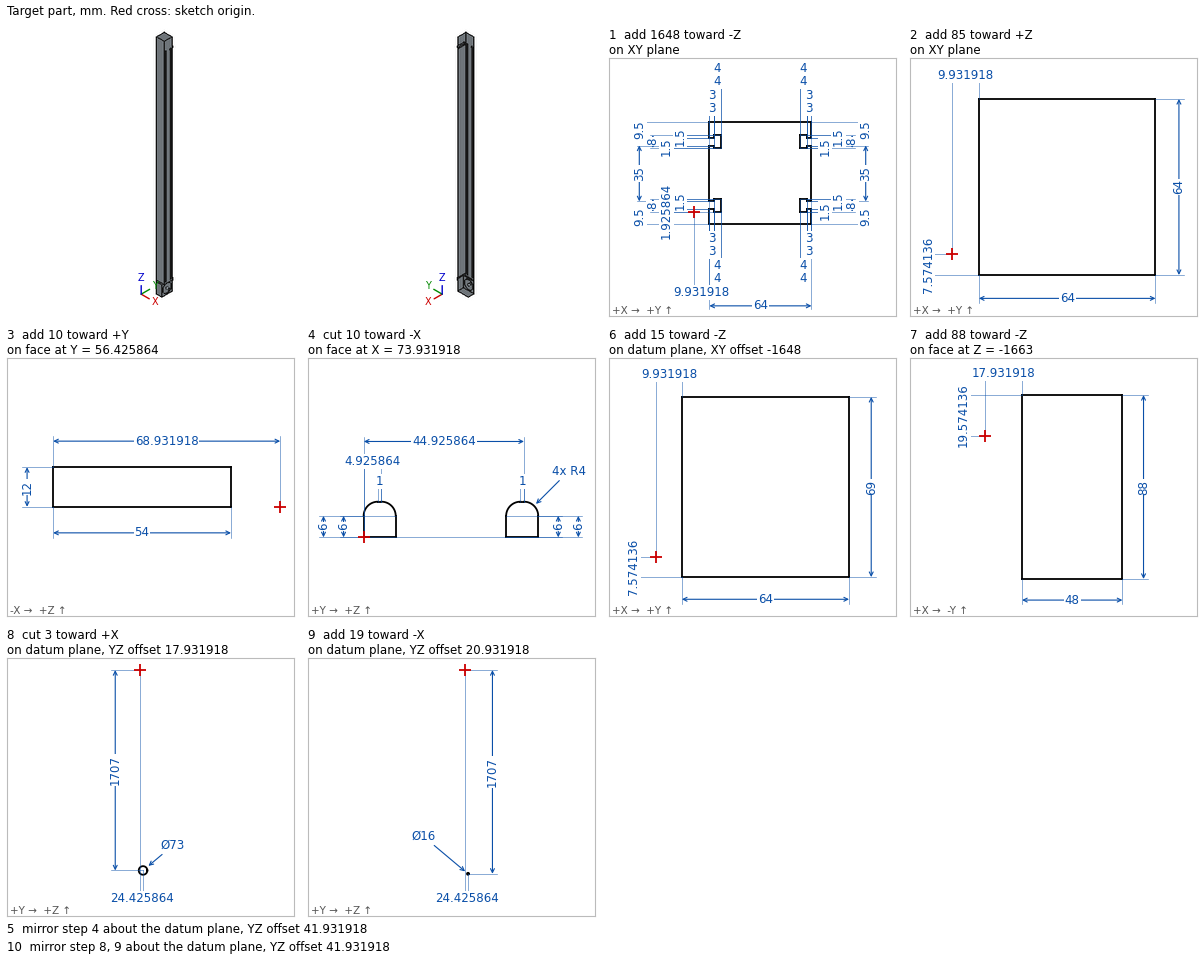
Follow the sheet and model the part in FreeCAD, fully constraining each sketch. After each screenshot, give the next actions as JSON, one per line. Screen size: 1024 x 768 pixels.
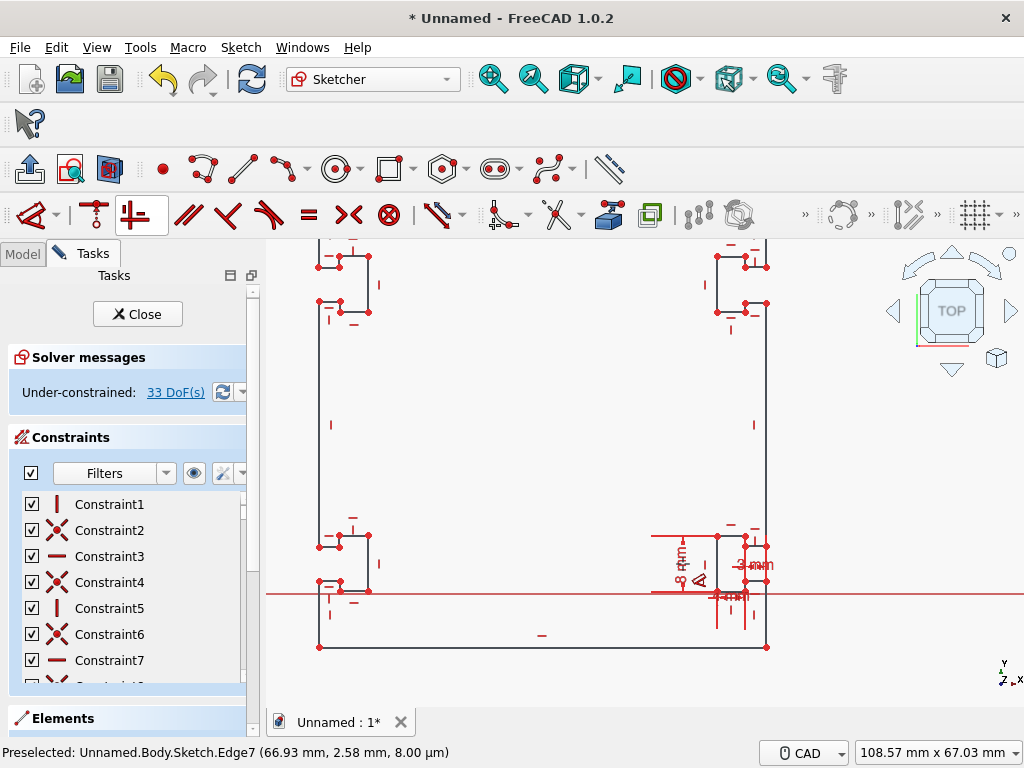
{"action": "scroll", "coordinate": [728, 536], "scroll_direction": "up", "scroll_amount": 2}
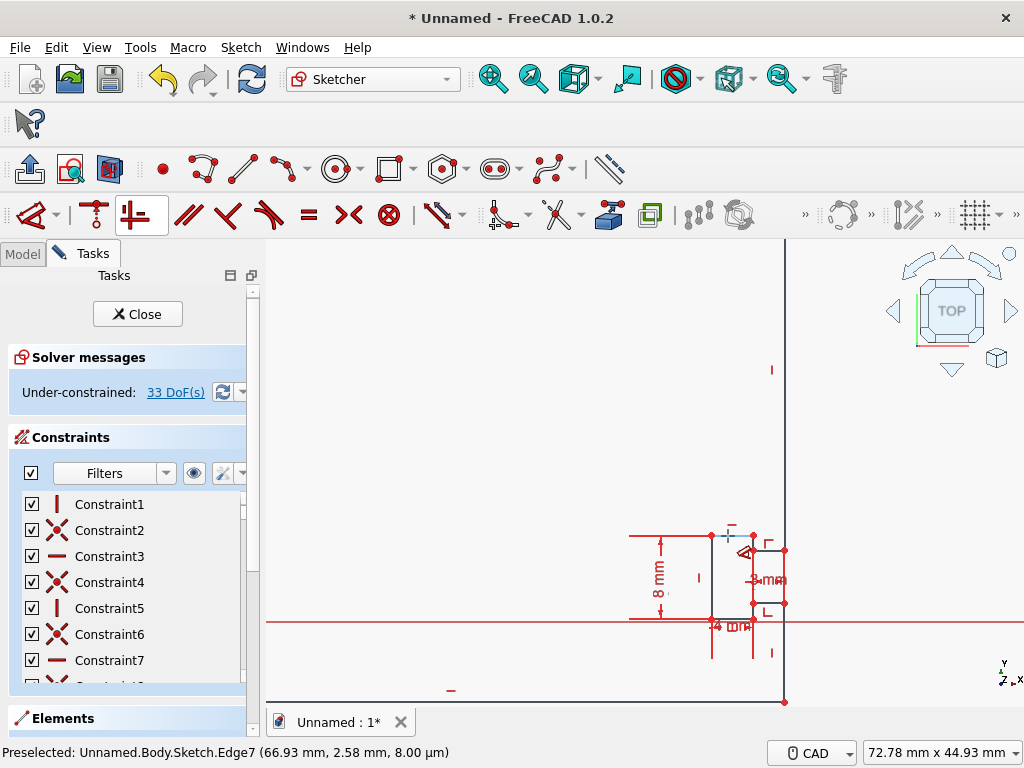
{"action": "left_click", "coordinate": [728, 536]}
{"action": "left_click", "coordinate": [732, 502]}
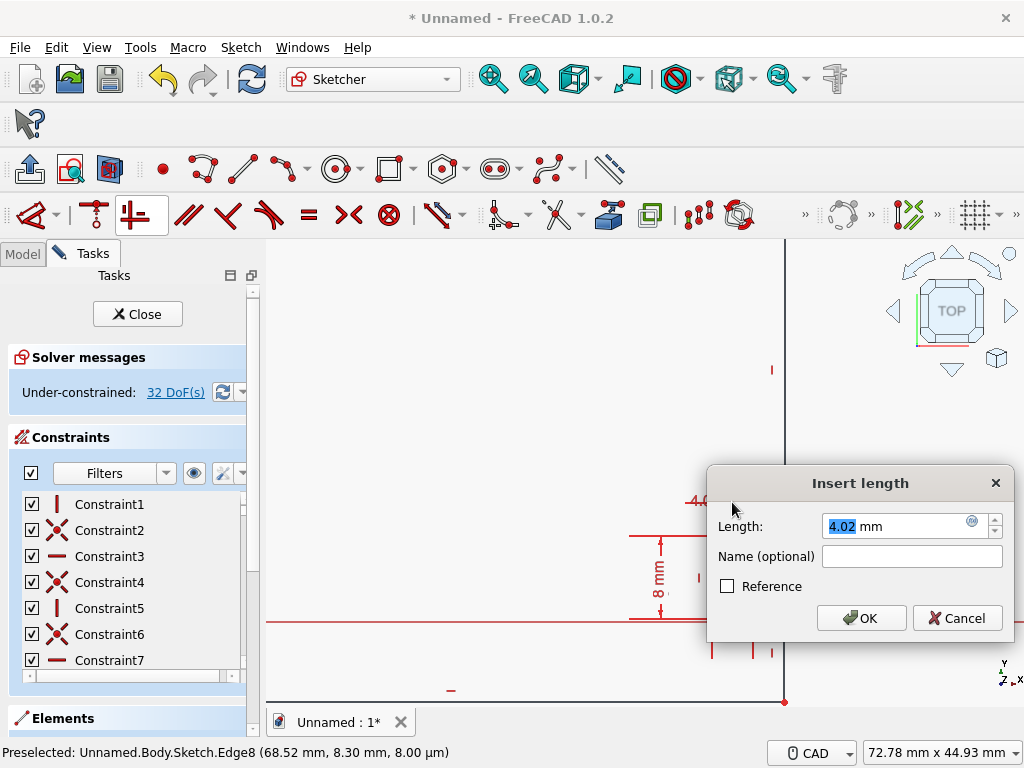
{"action": "type", "text": "4"}
{"action": "key", "text": "Return"}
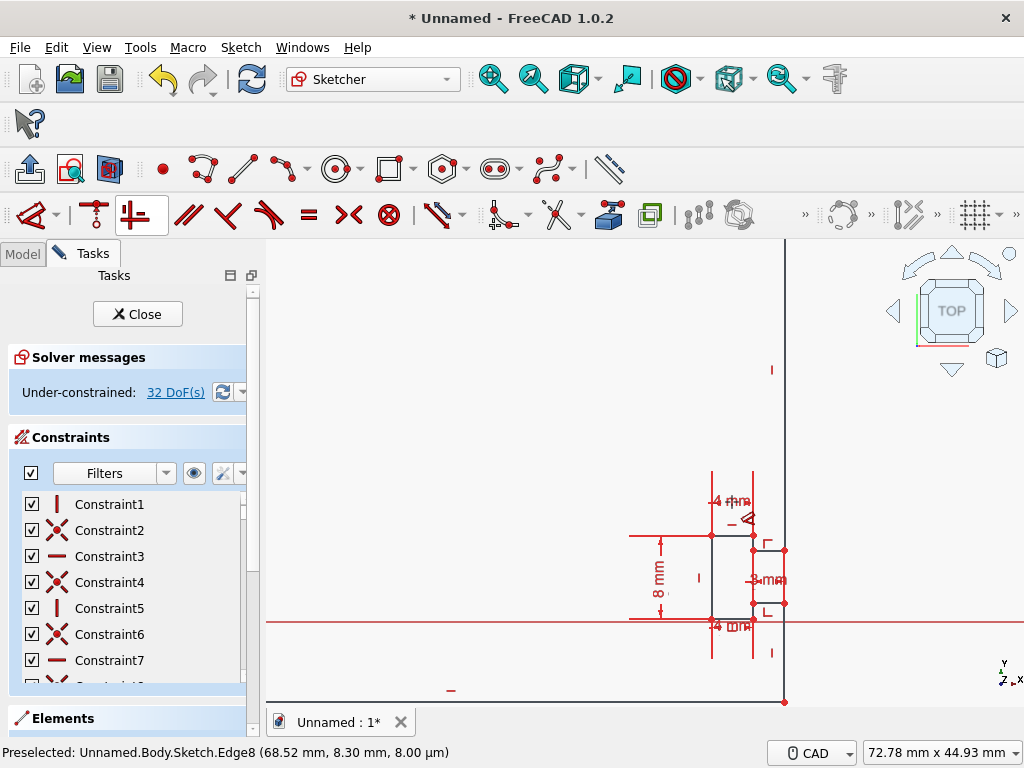
{"action": "scroll", "coordinate": [763, 551], "scroll_direction": "up", "scroll_amount": 2}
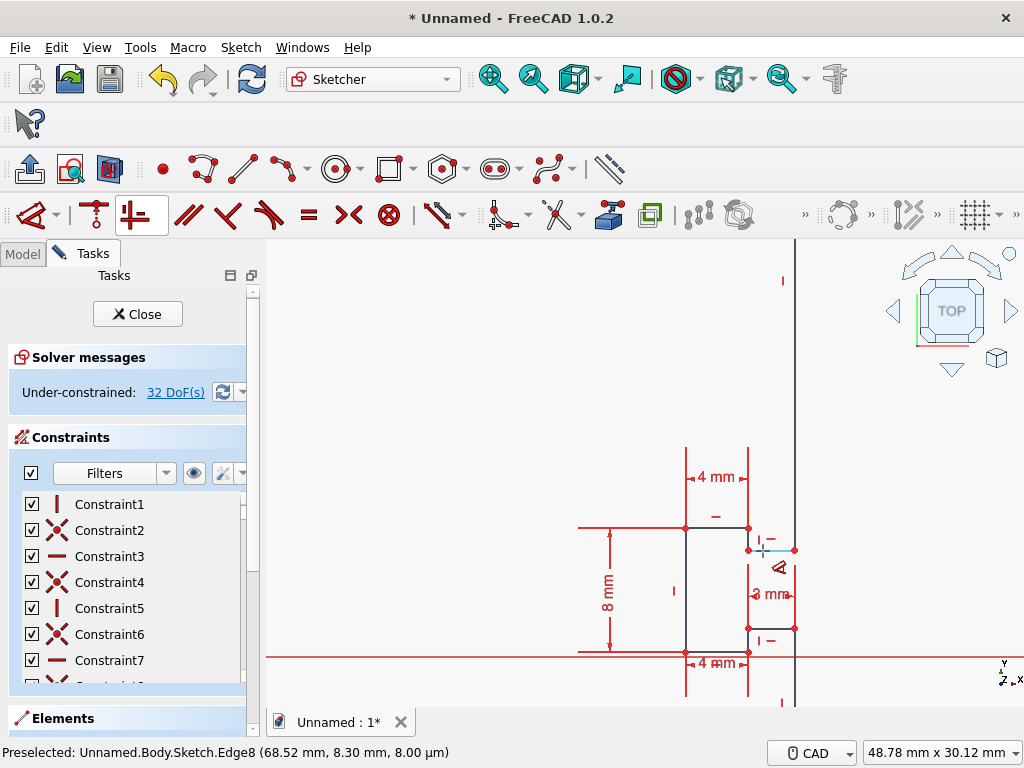
{"action": "left_click", "coordinate": [762, 551]}
{"action": "left_click", "coordinate": [771, 517]}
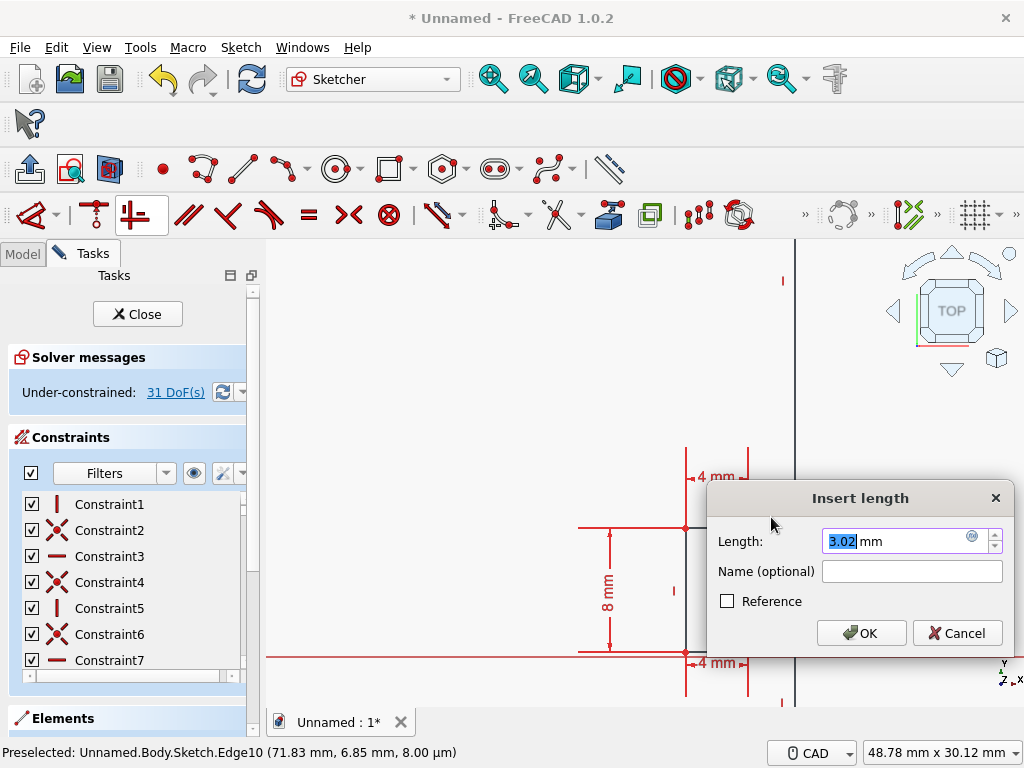
{"action": "type", "text": "3"}
{"action": "key", "text": "Return"}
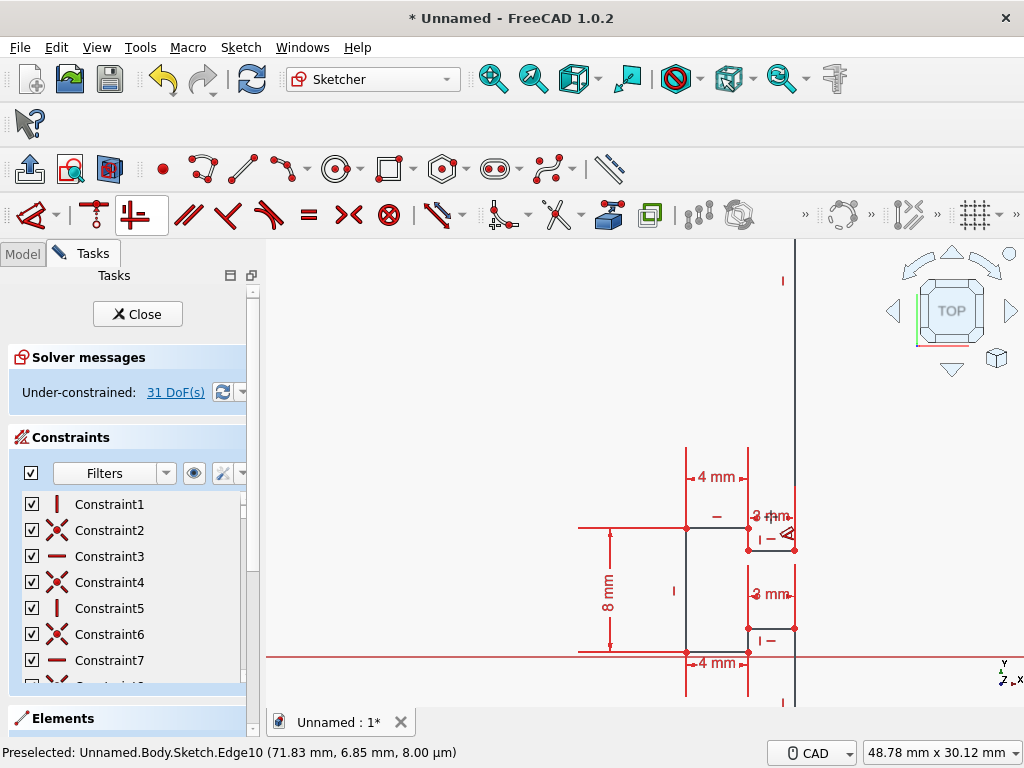
{"action": "scroll", "coordinate": [730, 557], "scroll_direction": "down", "scroll_amount": 6}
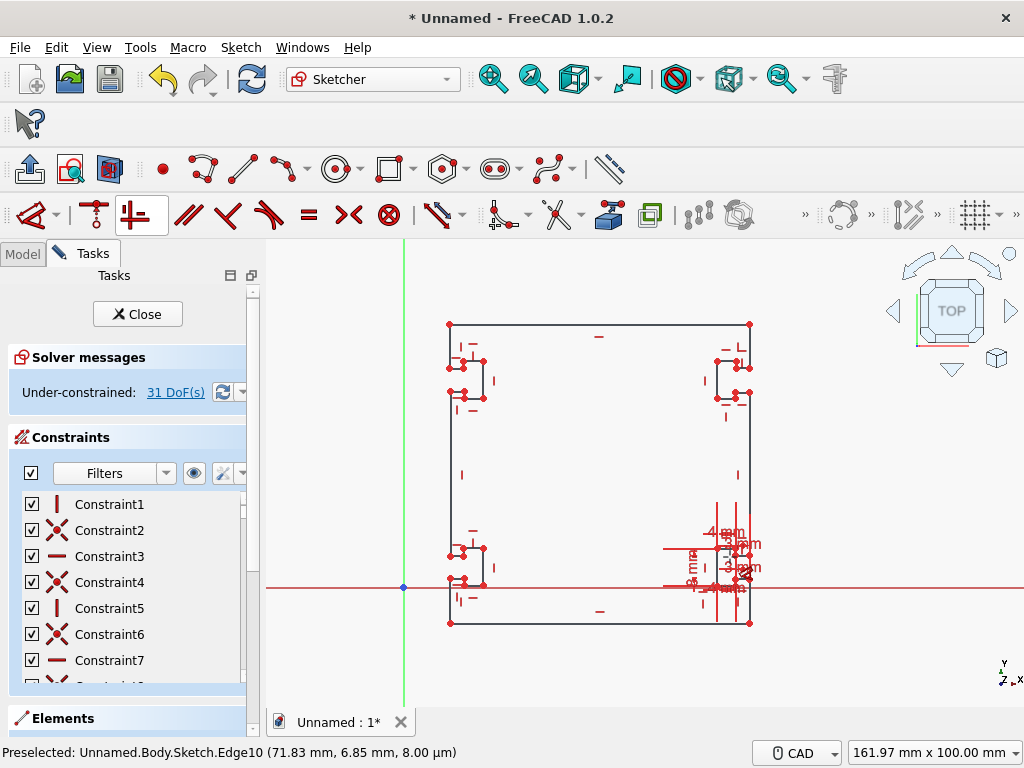
{"action": "scroll", "coordinate": [746, 393], "scroll_direction": "up", "scroll_amount": 6}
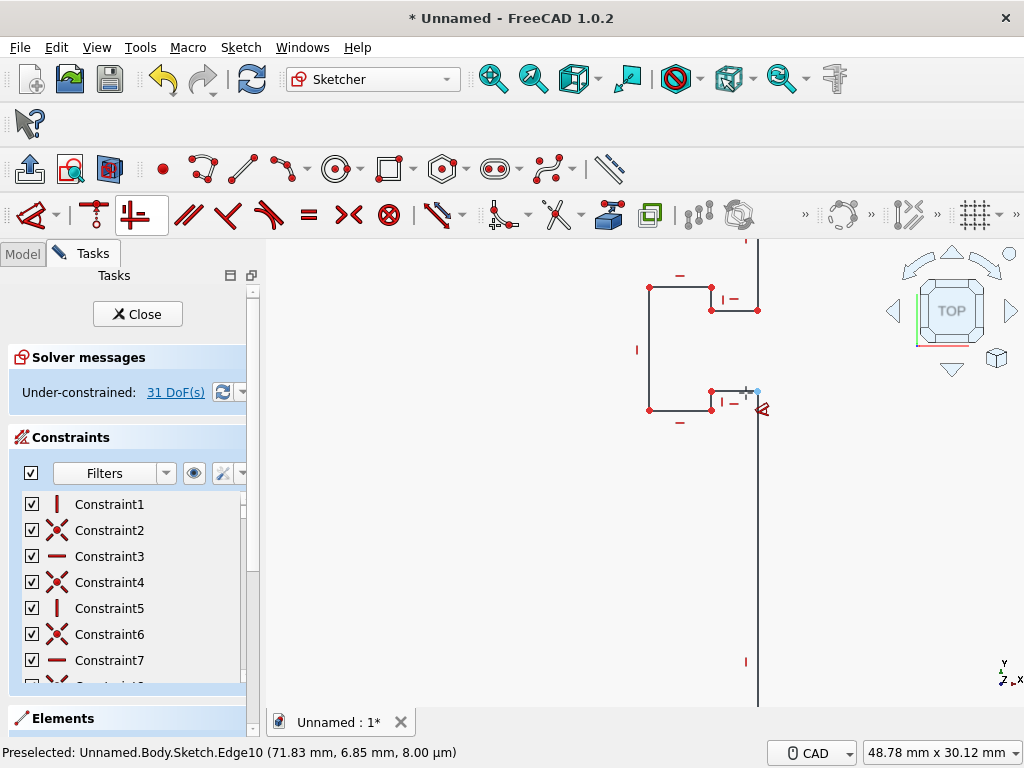
{"action": "left_click", "coordinate": [744, 391]}
{"action": "left_click", "coordinate": [735, 357]}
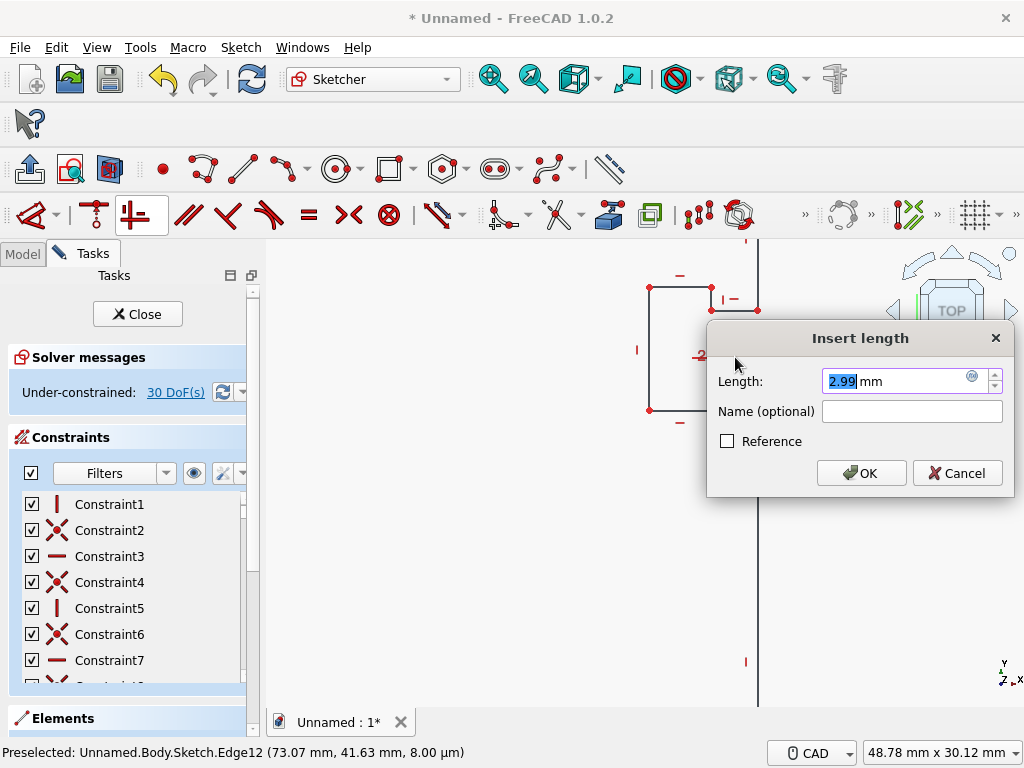
{"action": "type", "text": "3"}
{"action": "key", "text": "Return"}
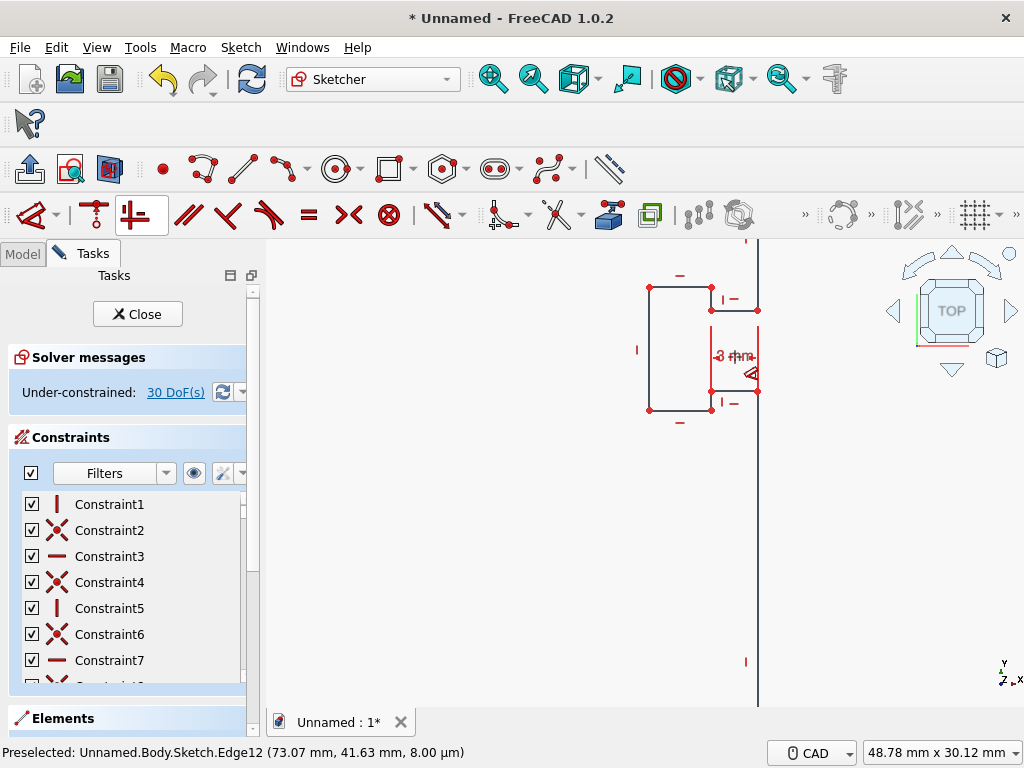
{"action": "left_click", "coordinate": [693, 411]}
{"action": "left_click", "coordinate": [680, 445]}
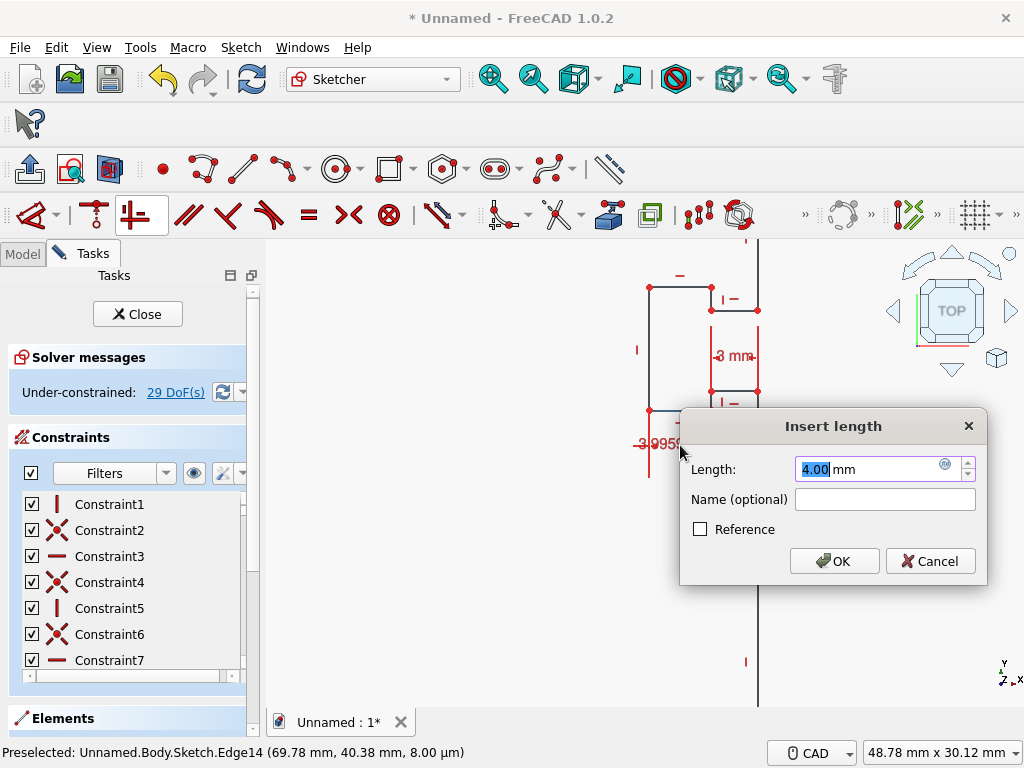
{"action": "type", "text": "4"}
{"action": "key", "text": "Return"}